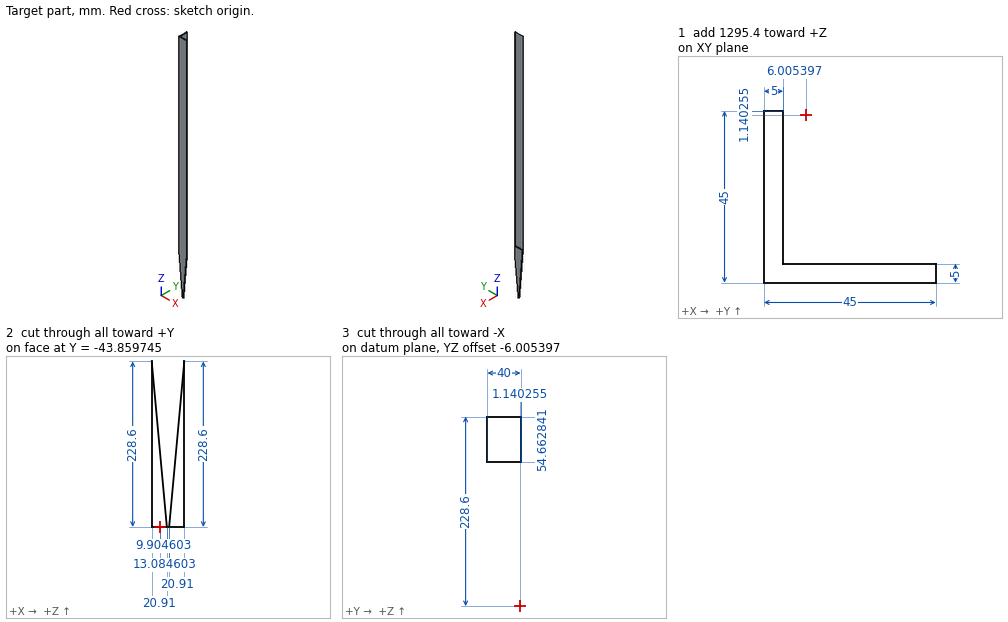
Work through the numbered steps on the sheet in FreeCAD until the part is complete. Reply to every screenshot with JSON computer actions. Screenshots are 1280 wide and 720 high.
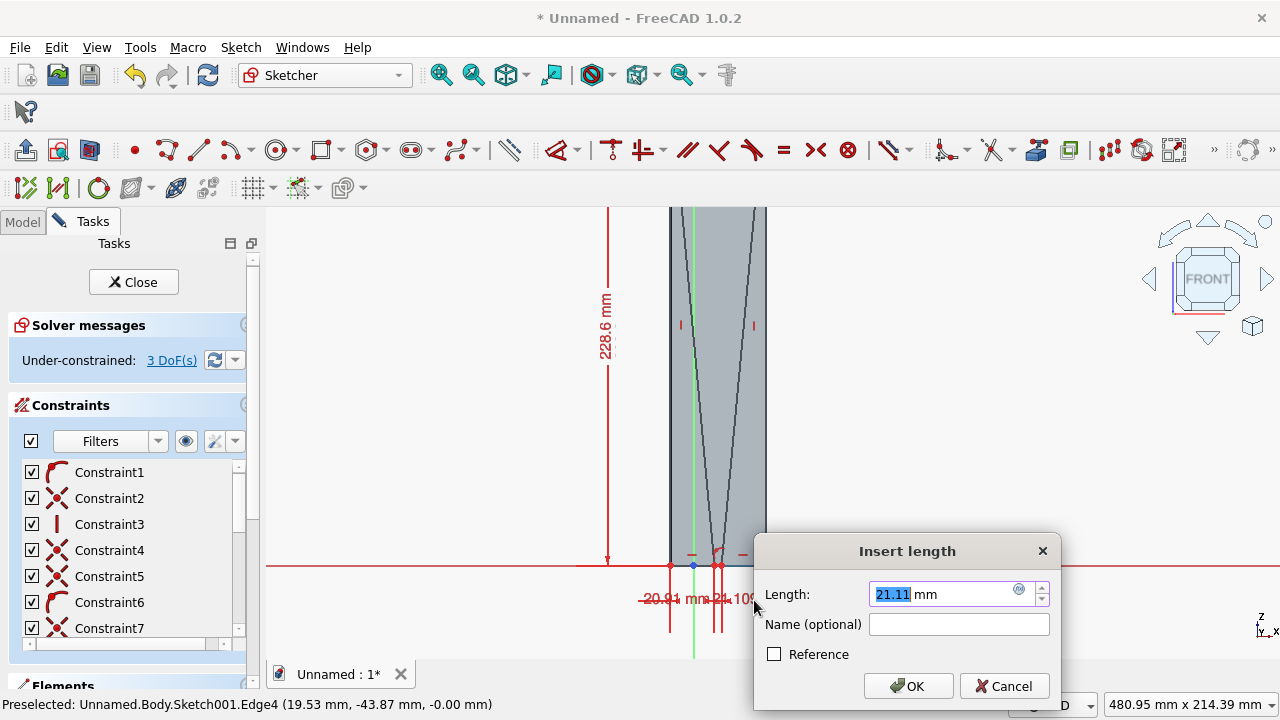
{"action": "type", "text": "20.91"}
{"action": "key", "text": "Return"}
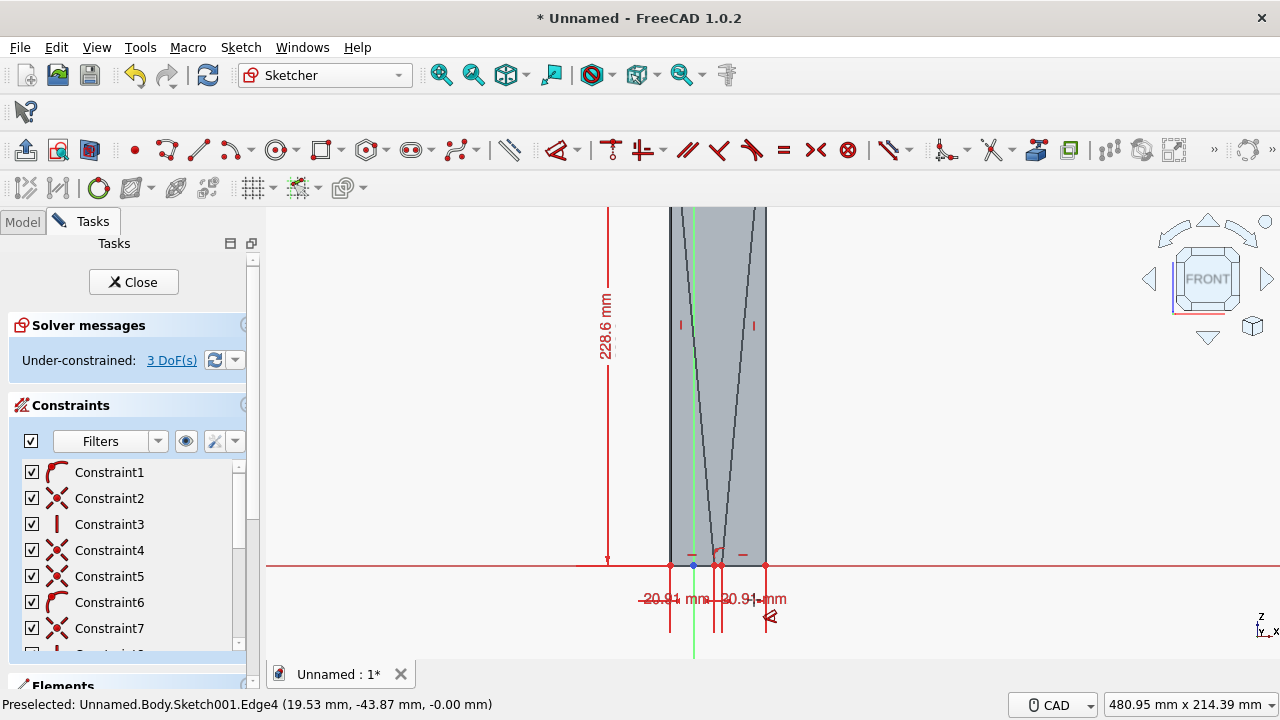
{"action": "left_click", "coordinate": [766, 422]}
{"action": "left_click", "coordinate": [800, 400]}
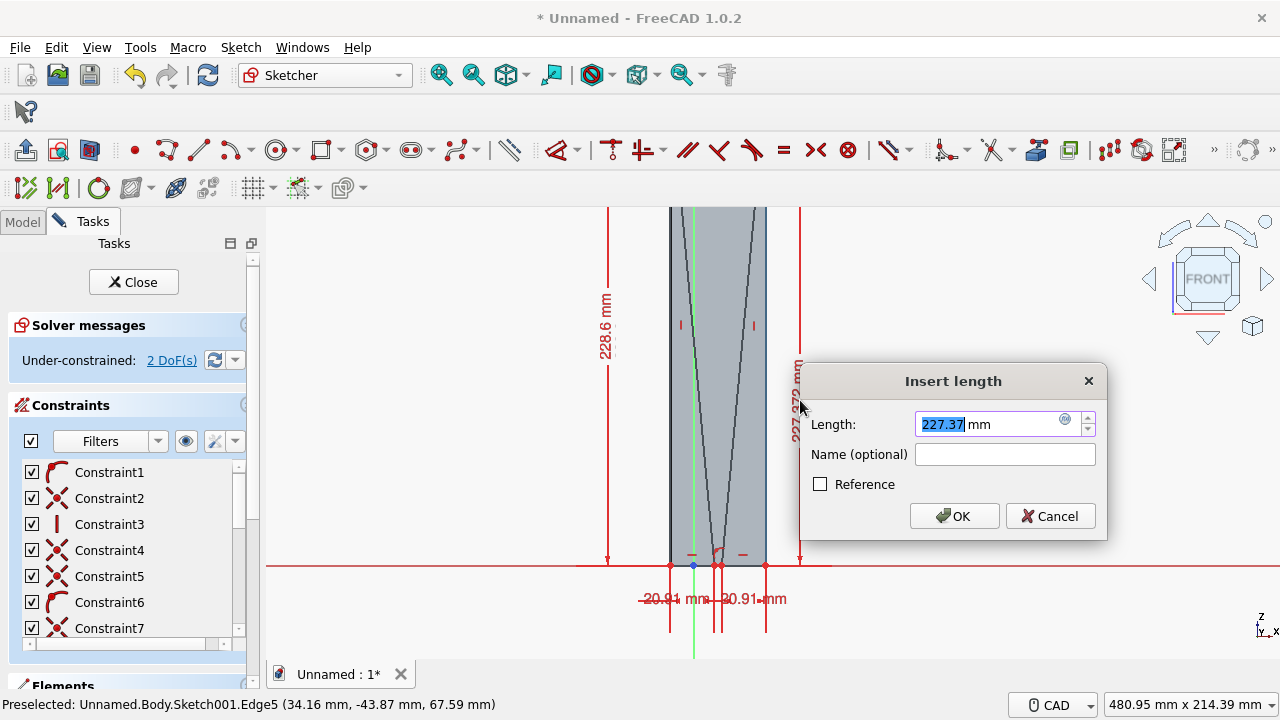
{"action": "type", "text": "228.6"}
{"action": "key", "text": "Return"}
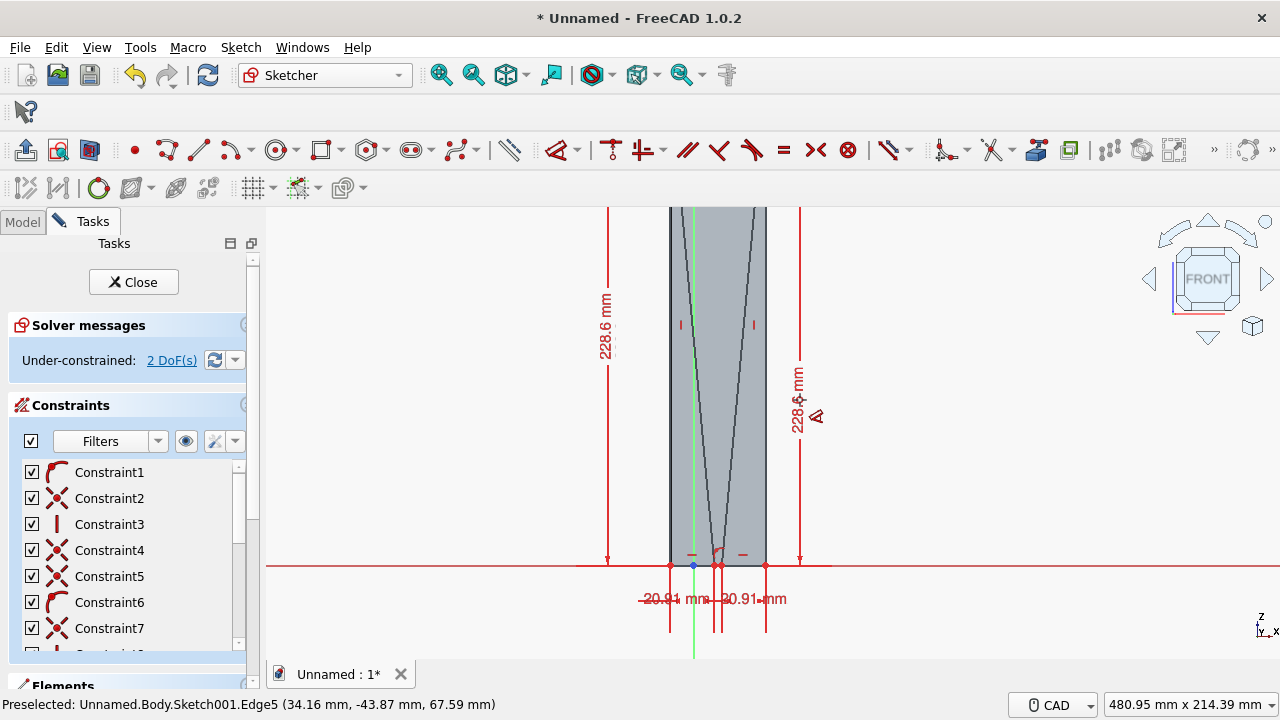
{"action": "scroll", "coordinate": [714, 566], "scroll_direction": "up", "scroll_amount": 4}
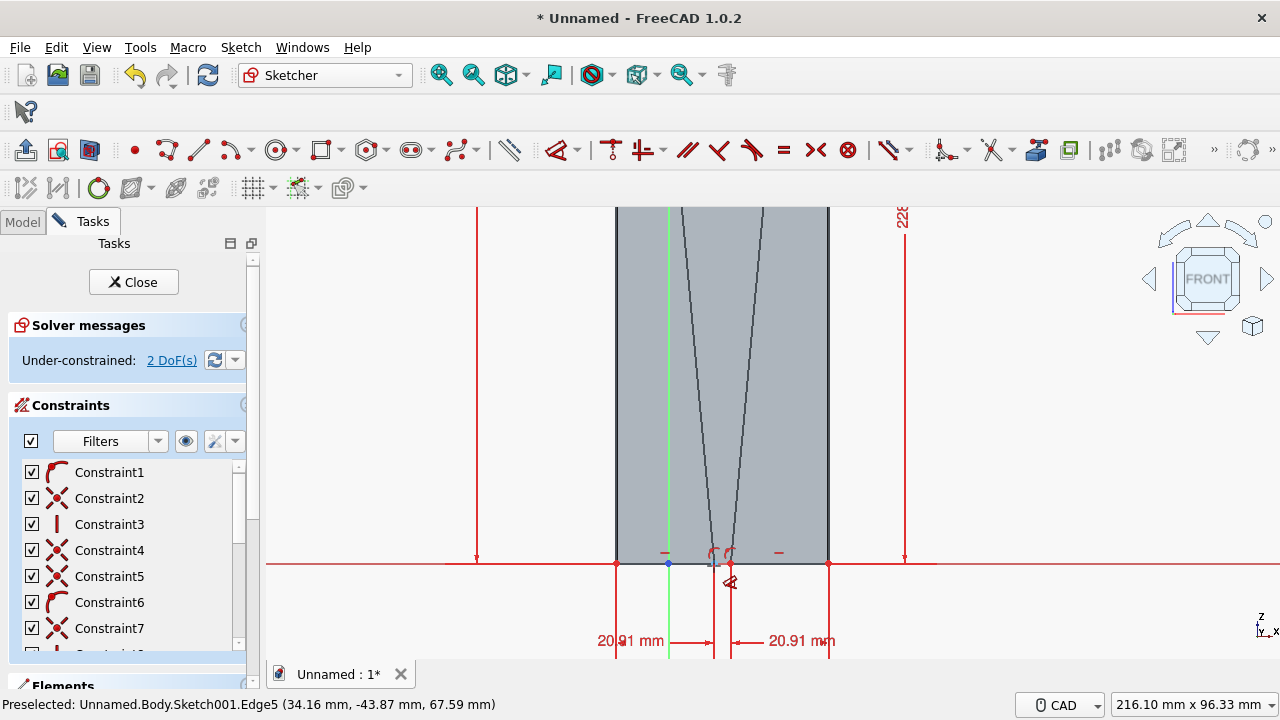
{"action": "left_click", "coordinate": [714, 564]}
{"action": "left_click", "coordinate": [692, 598]}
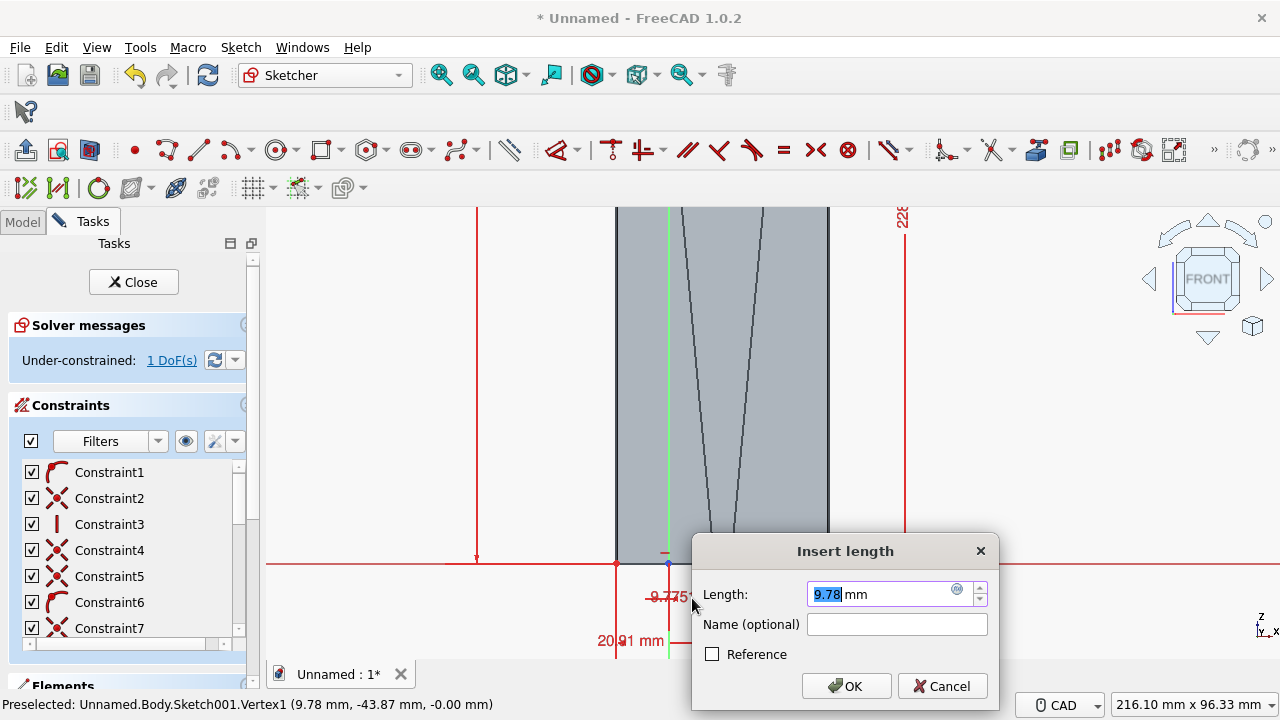
{"action": "type", "text": "9.904603"}
{"action": "key", "text": "Return"}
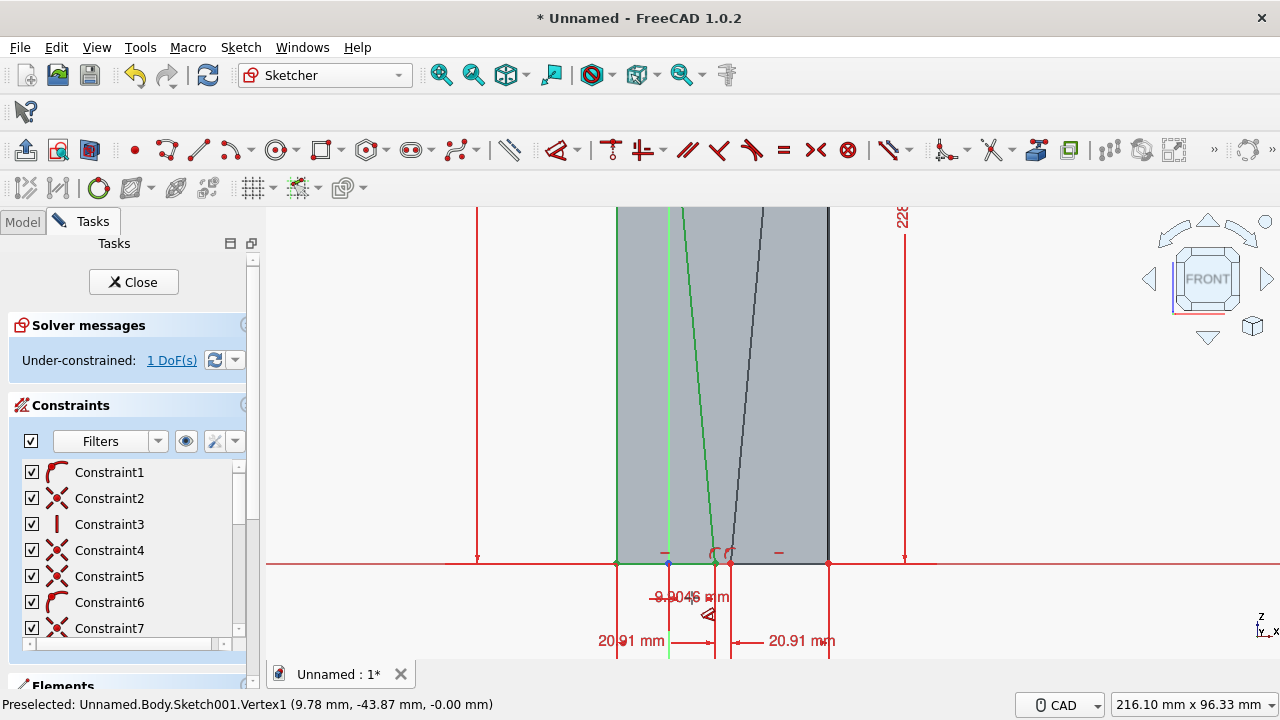
{"action": "left_click", "coordinate": [731, 564]}
{"action": "left_click", "coordinate": [685, 530]}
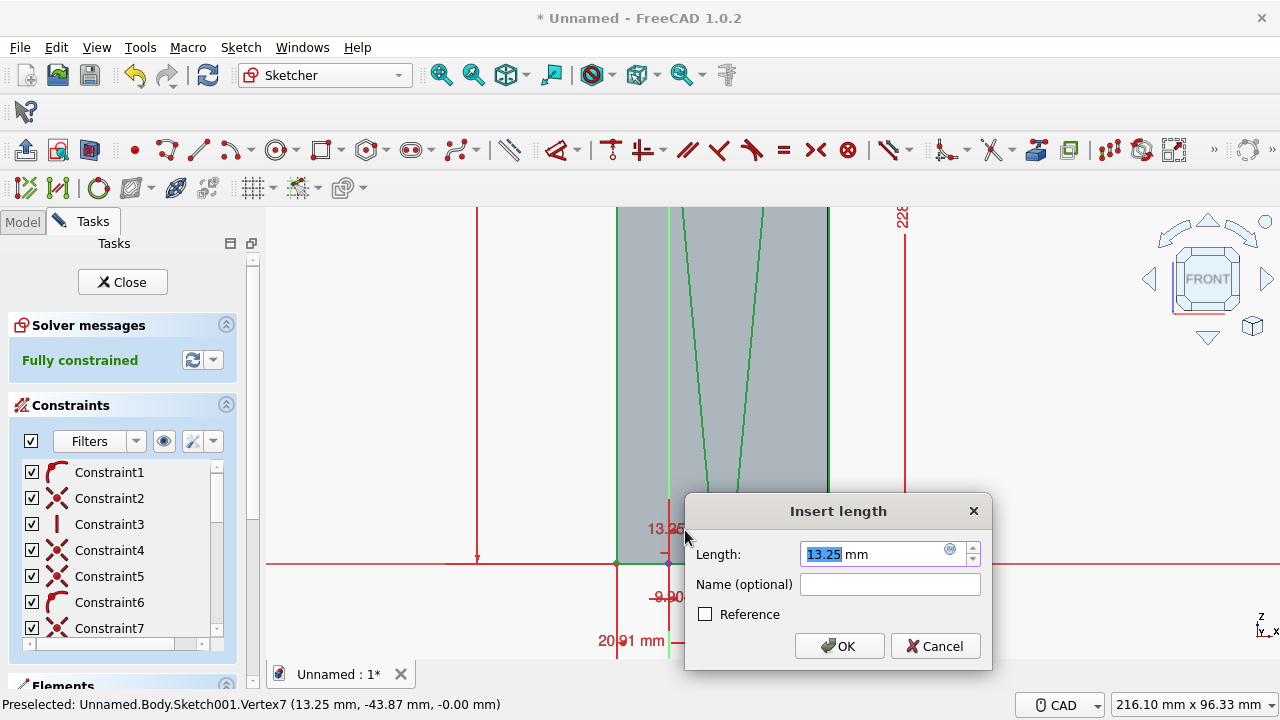
{"action": "type", "text": "13.084603"}
{"action": "key", "text": "Return"}
{"action": "key", "text": "Escape"}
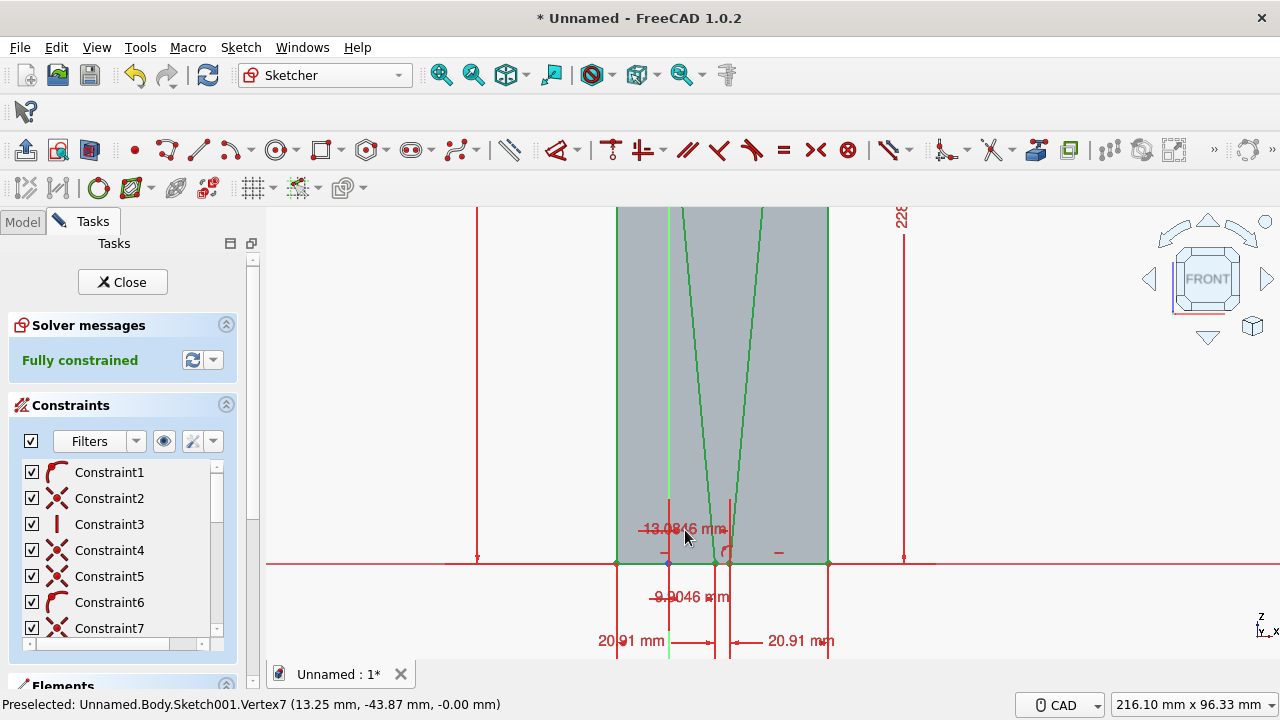
{"action": "left_click", "coordinate": [123, 282]}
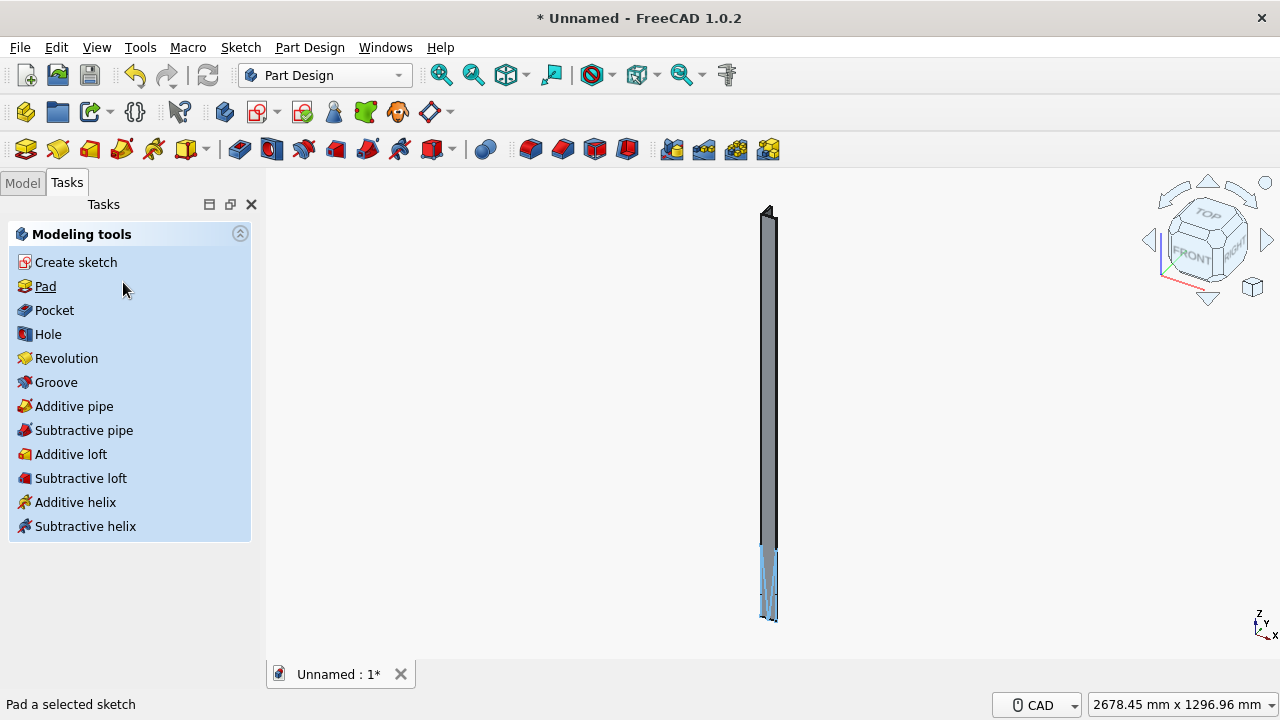
{"action": "left_click", "coordinate": [240, 150]}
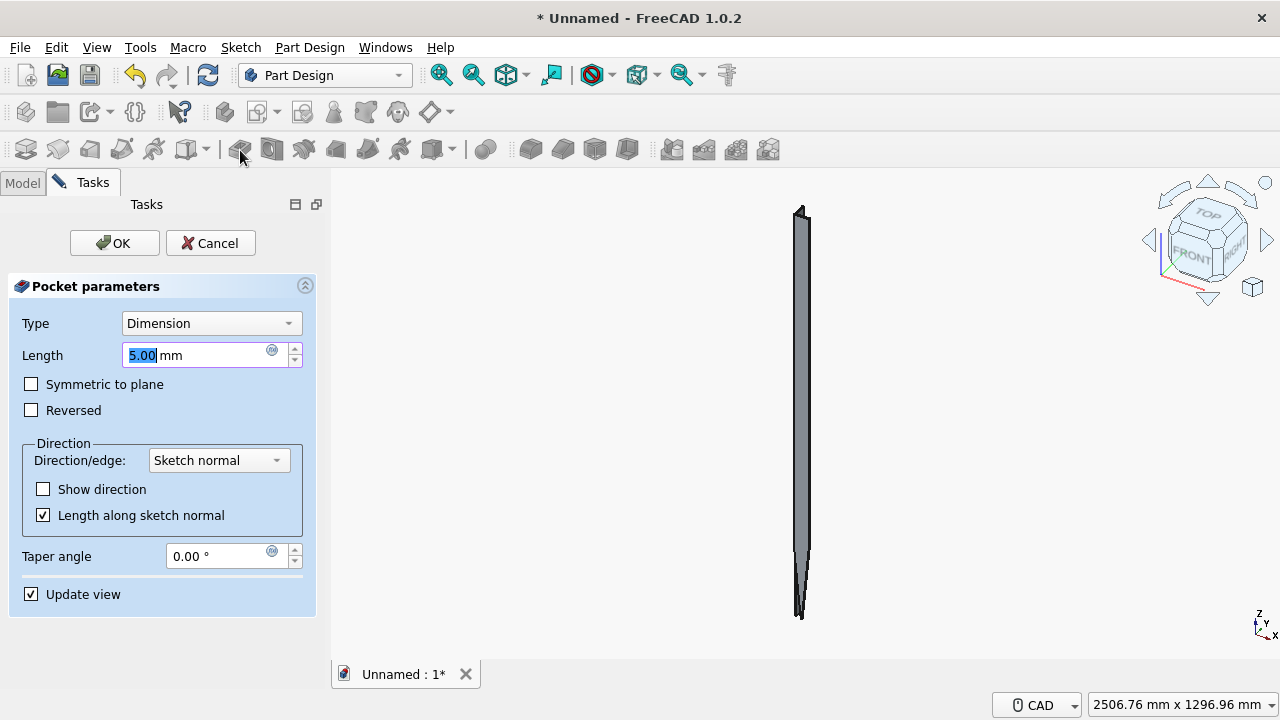
{"action": "left_click", "coordinate": [212, 324]}